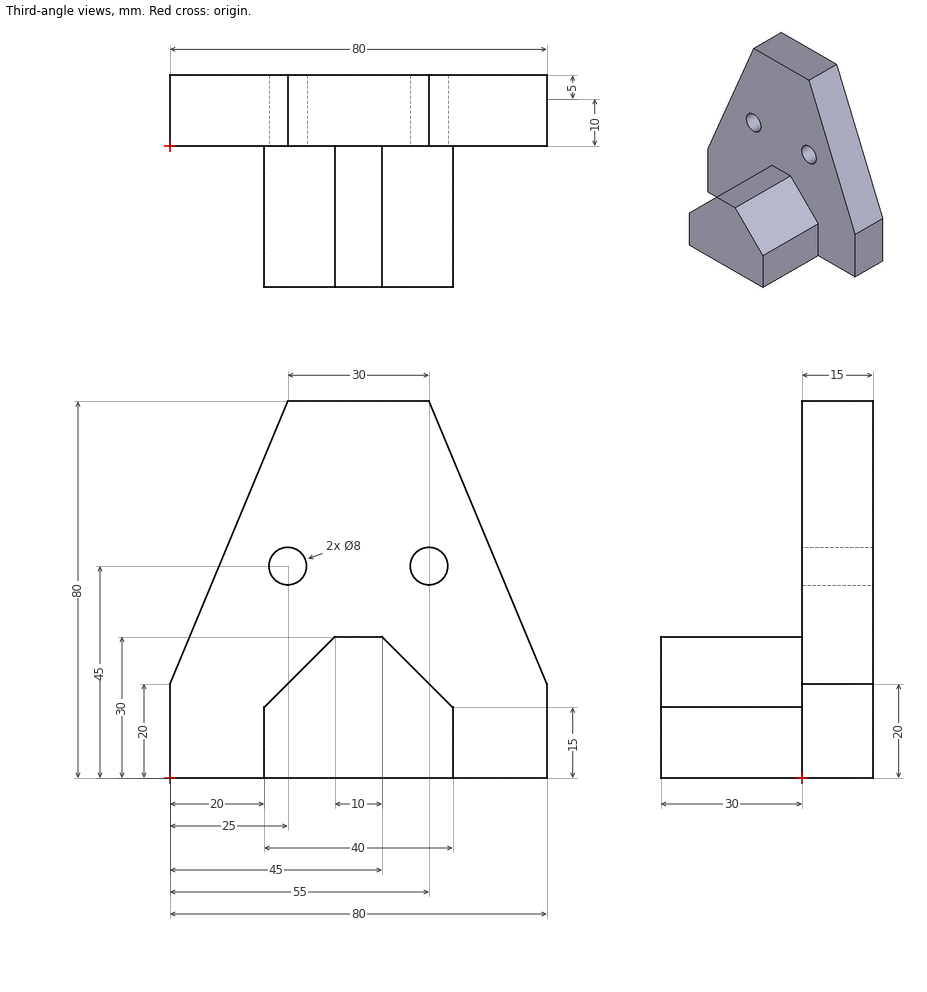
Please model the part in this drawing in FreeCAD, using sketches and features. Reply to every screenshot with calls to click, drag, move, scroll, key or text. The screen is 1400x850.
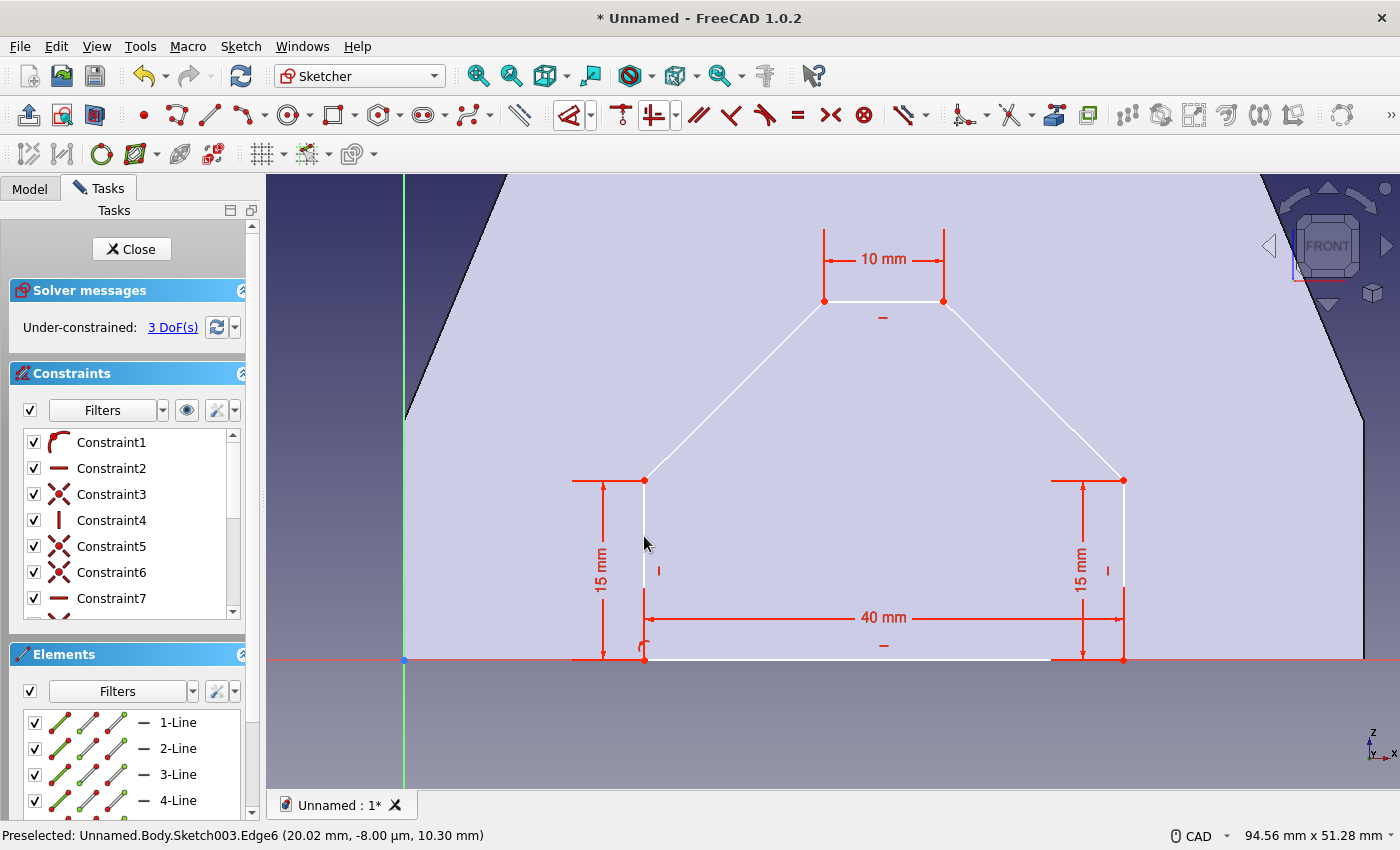
click(644, 660)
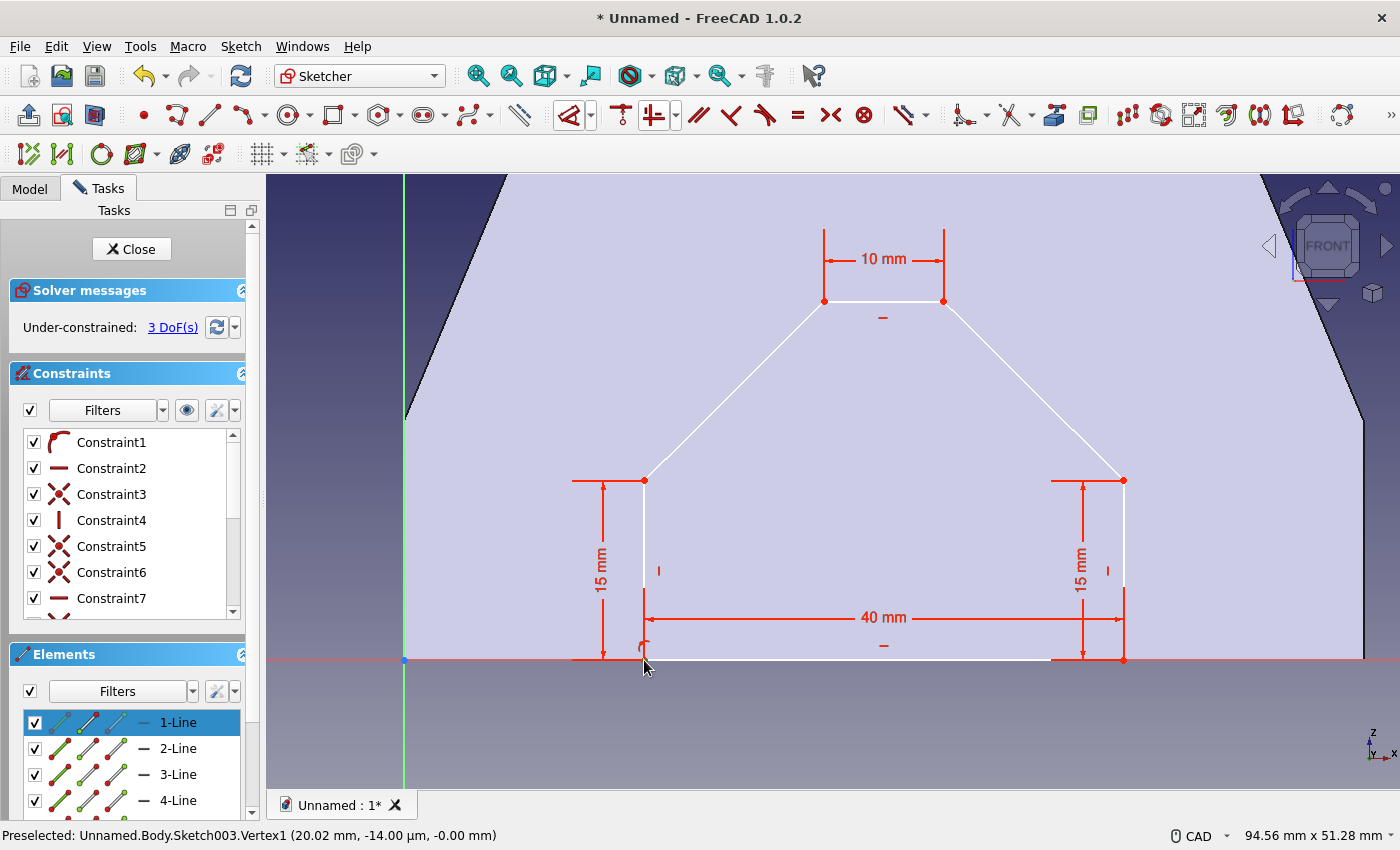
key(l)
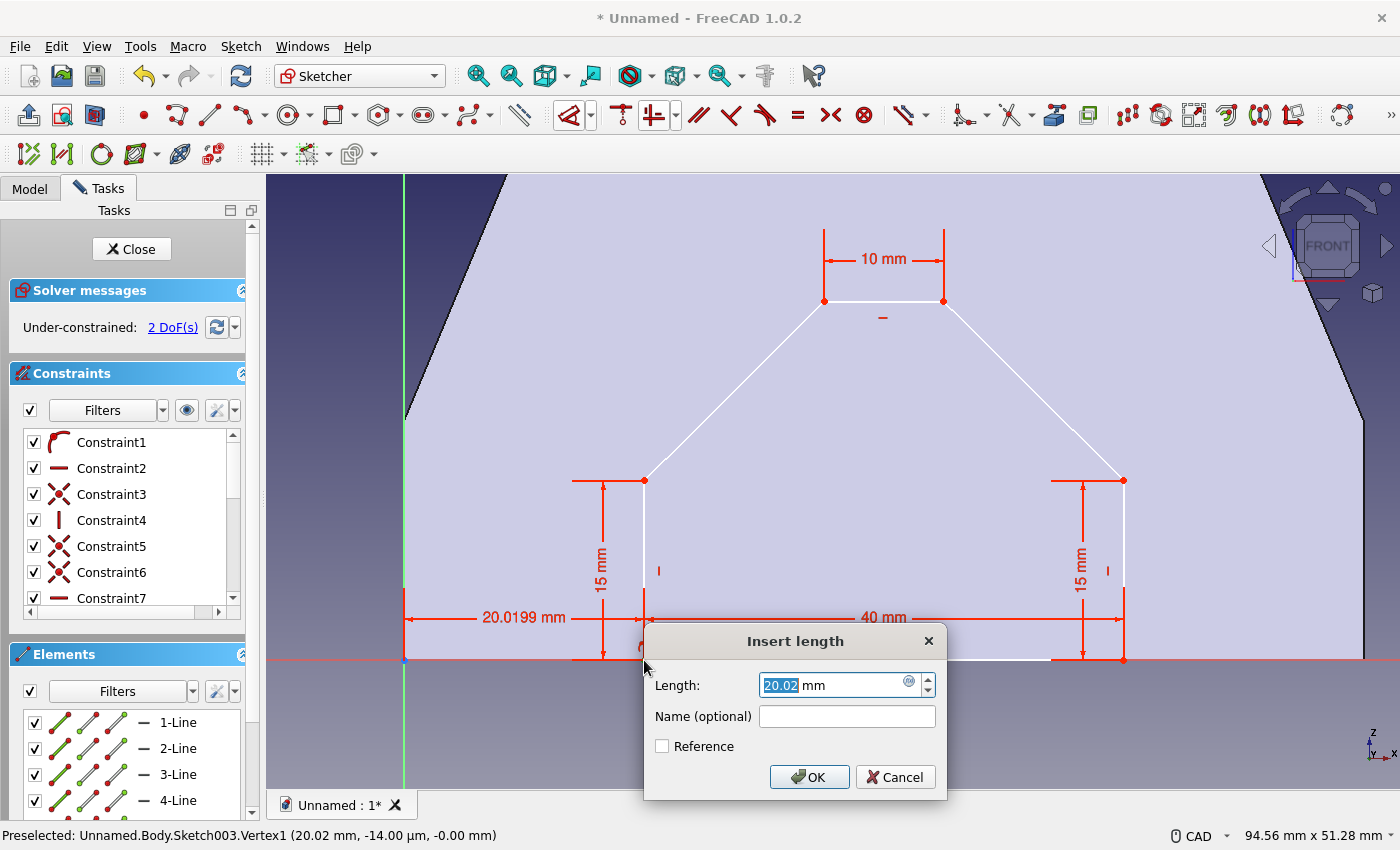
text(20)
key(Return)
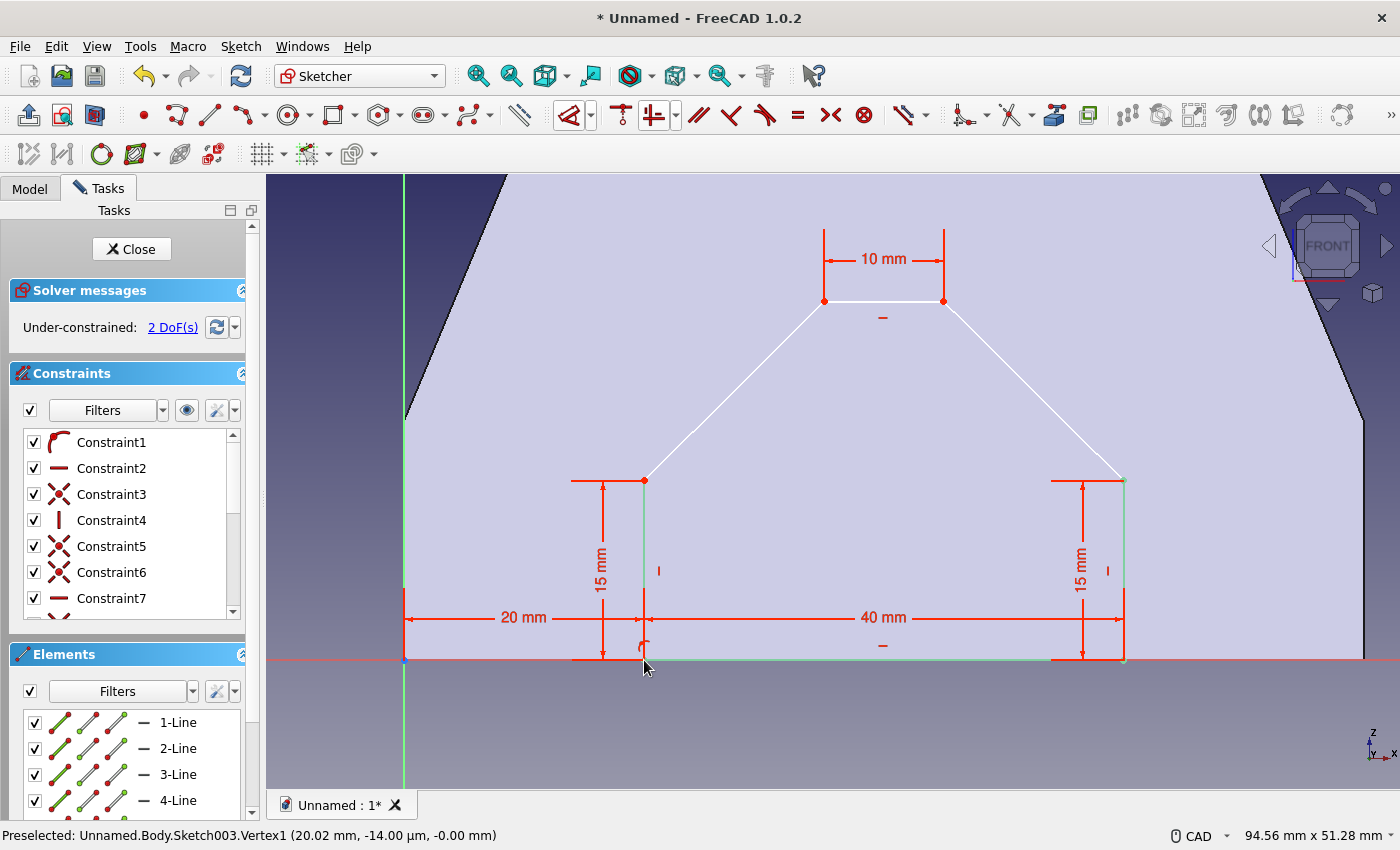
click(944, 302)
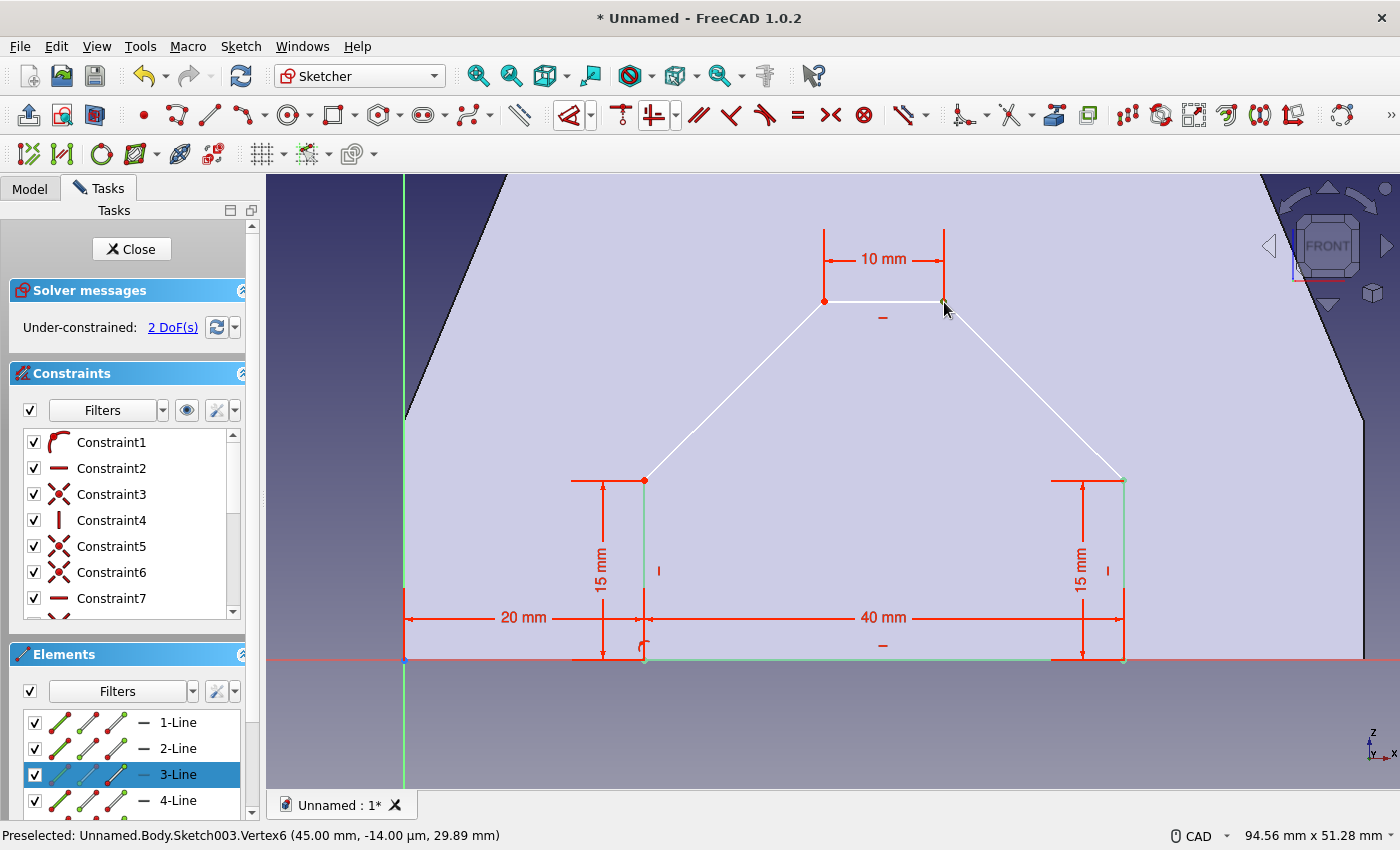
click(590, 116)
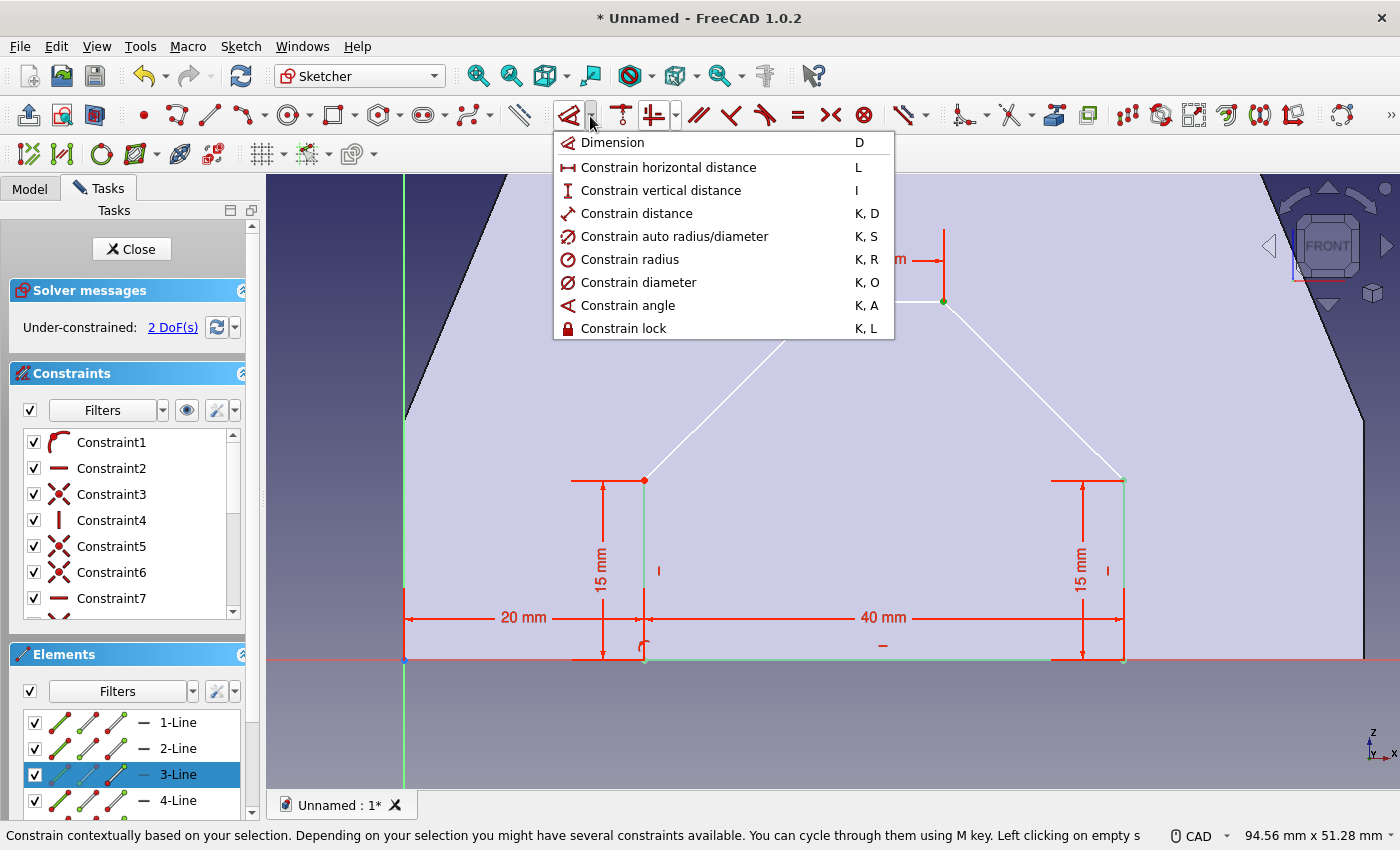
click(724, 168)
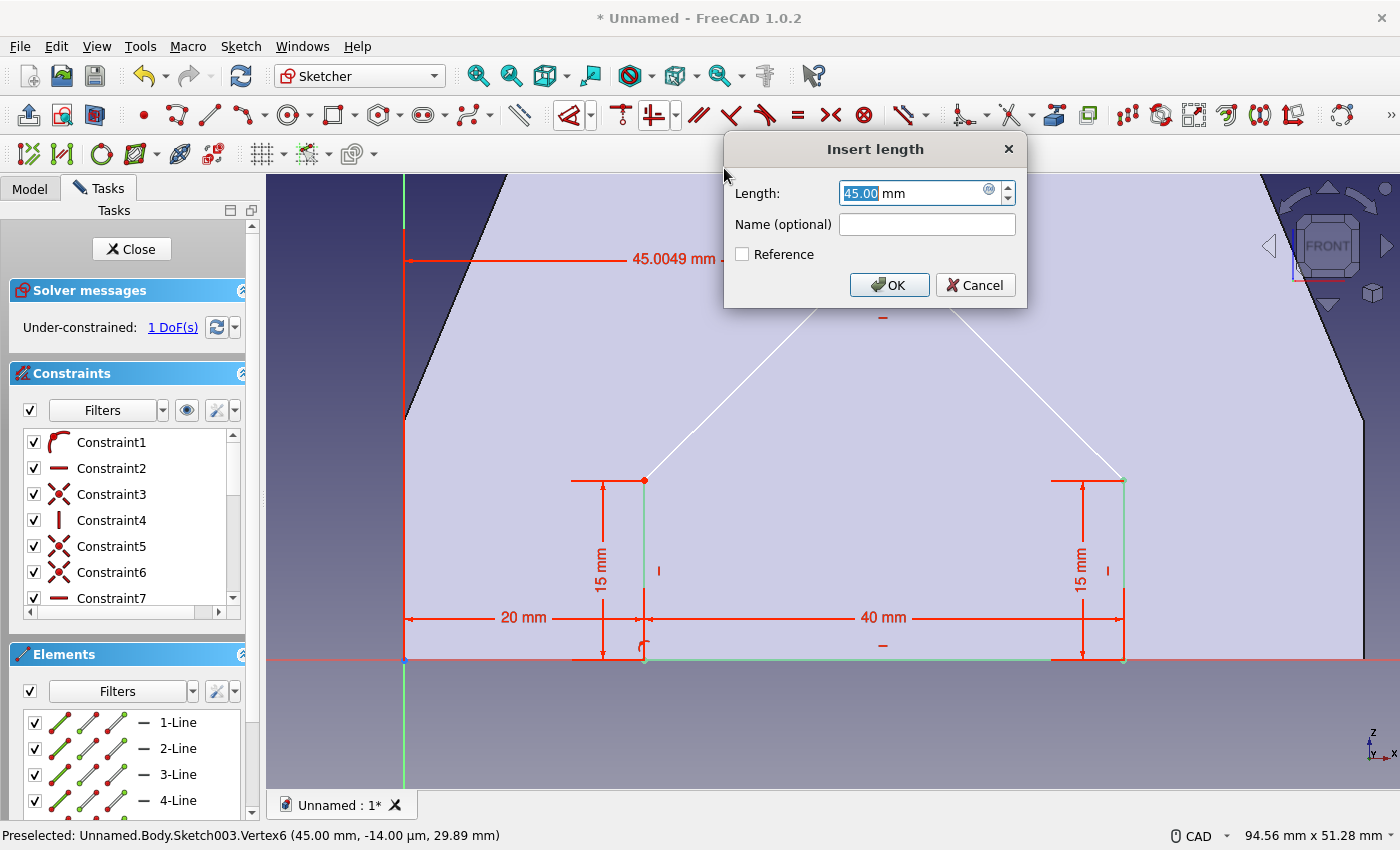
text(45)
key(Return)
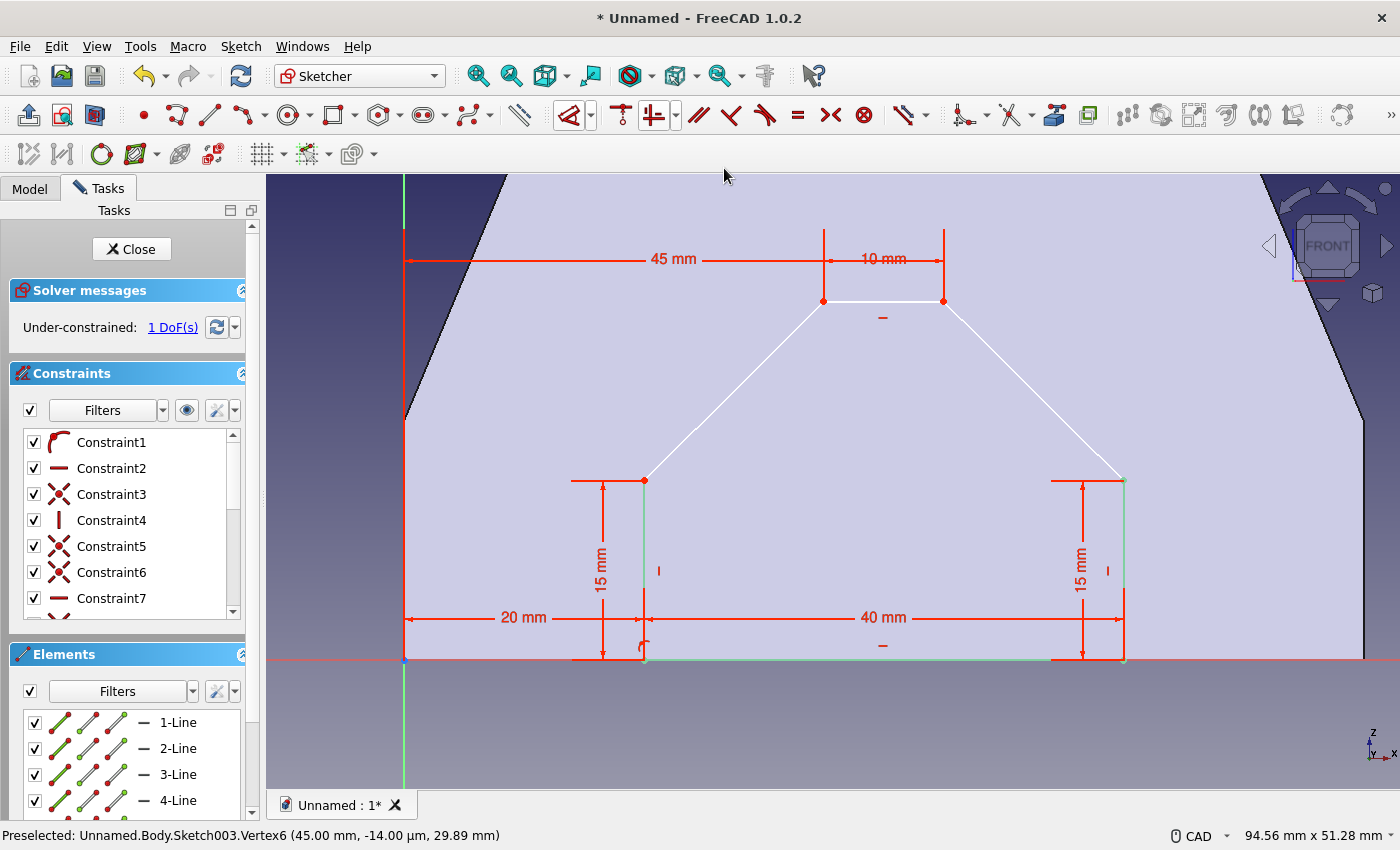
click(944, 302)